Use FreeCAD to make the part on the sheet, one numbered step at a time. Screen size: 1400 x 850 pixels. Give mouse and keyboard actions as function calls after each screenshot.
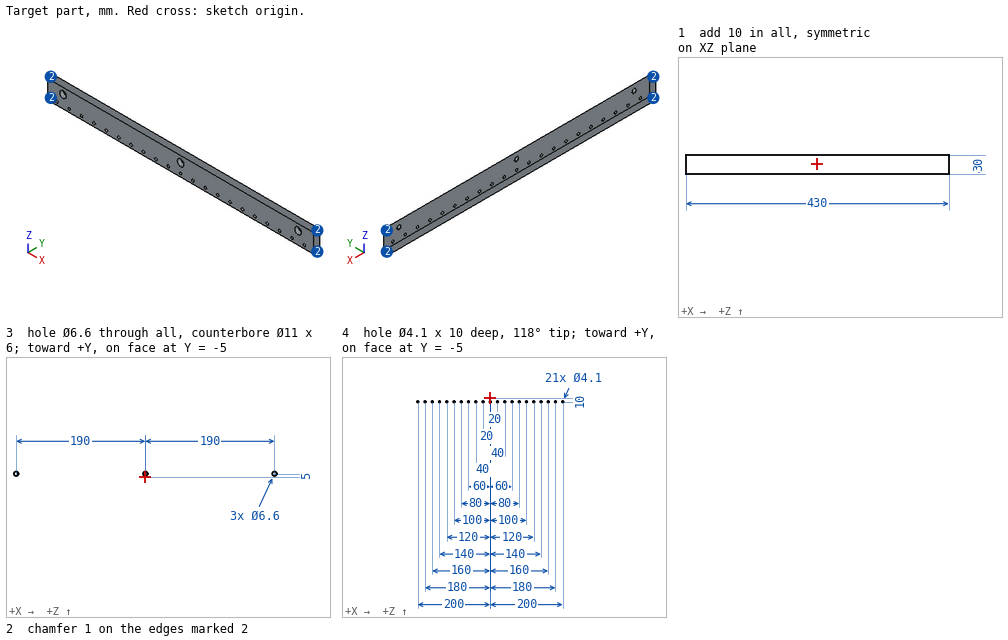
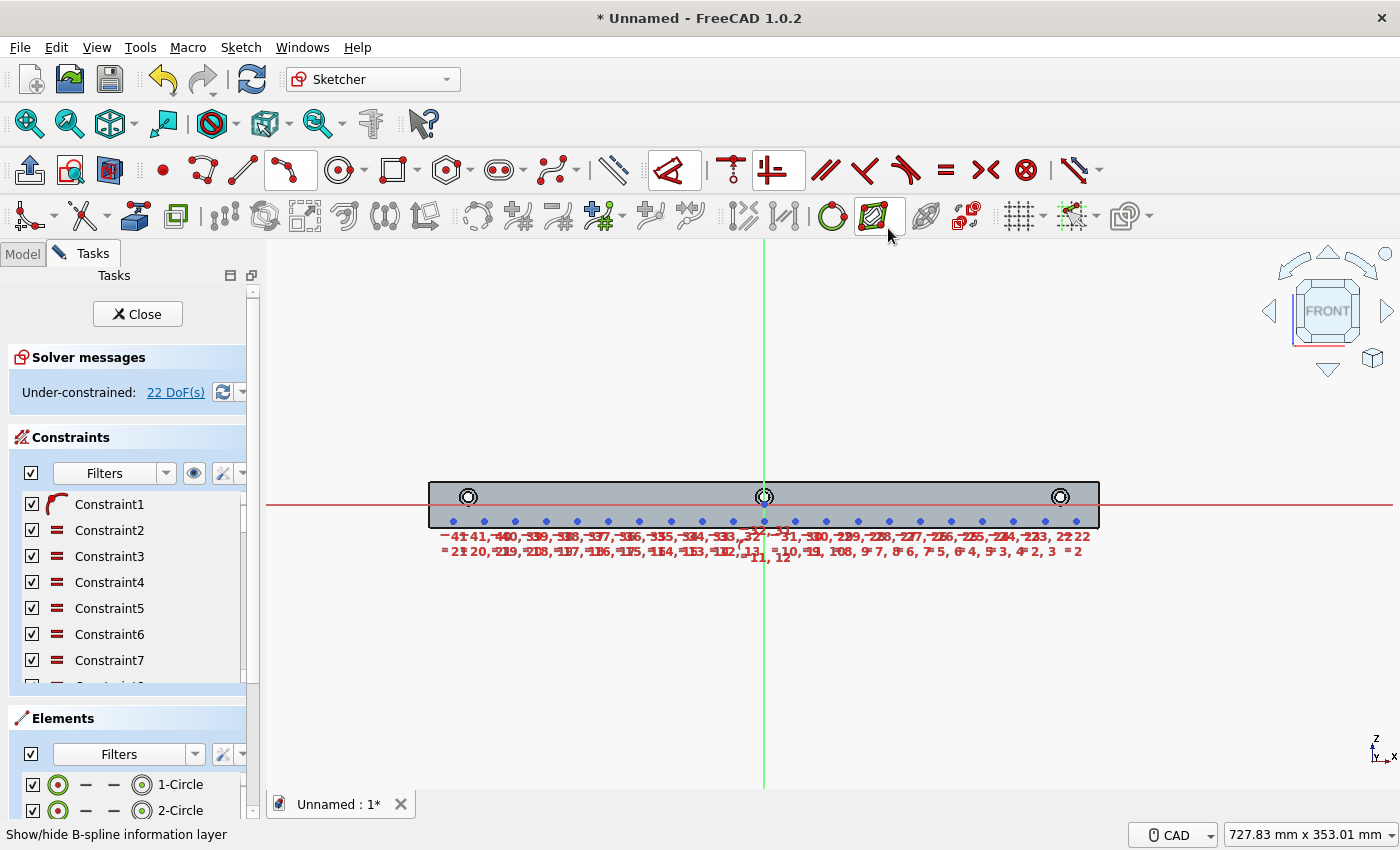
scroll(1074, 522, up, 10)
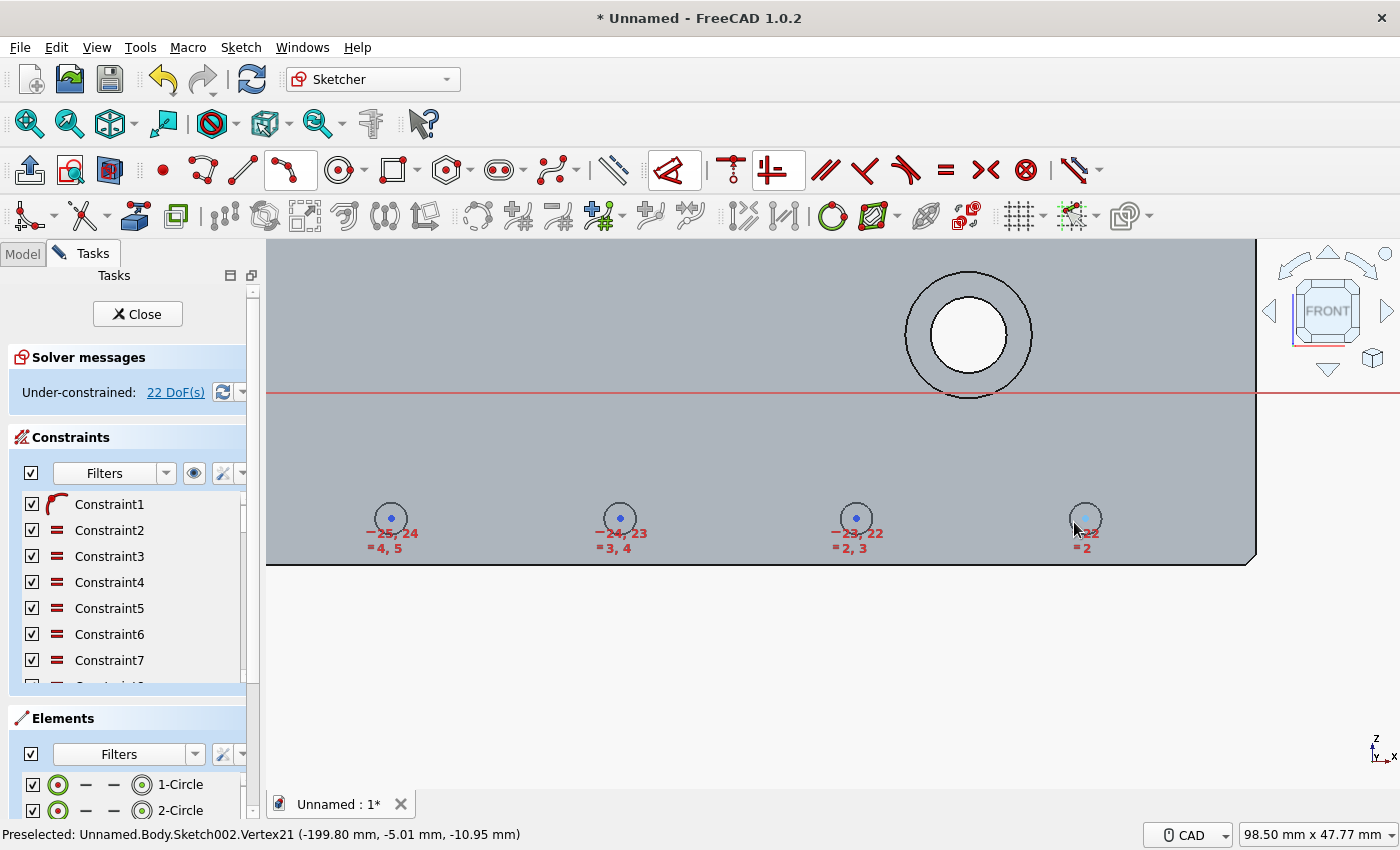
click(1070, 518)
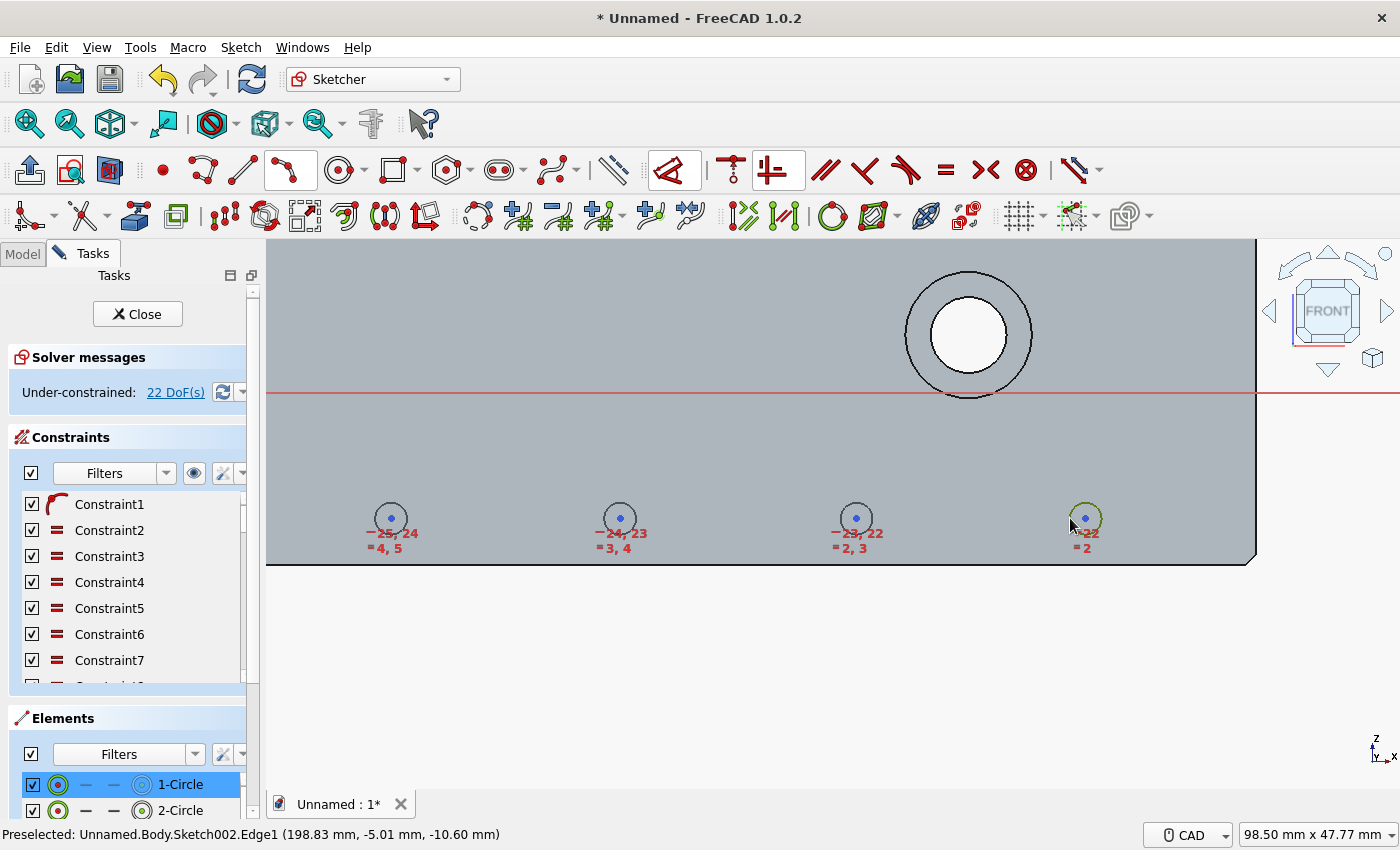
click(696, 170)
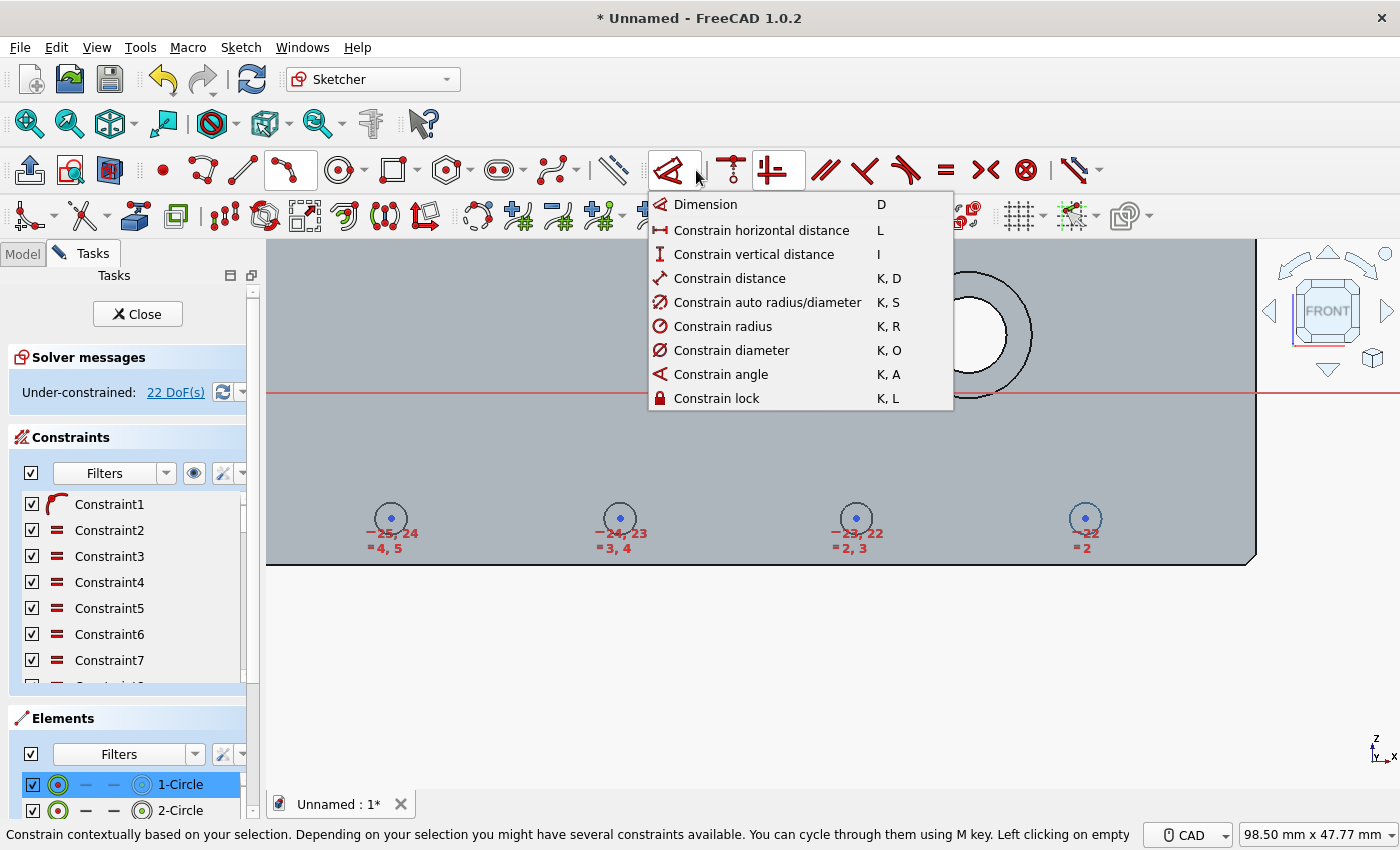
click(801, 350)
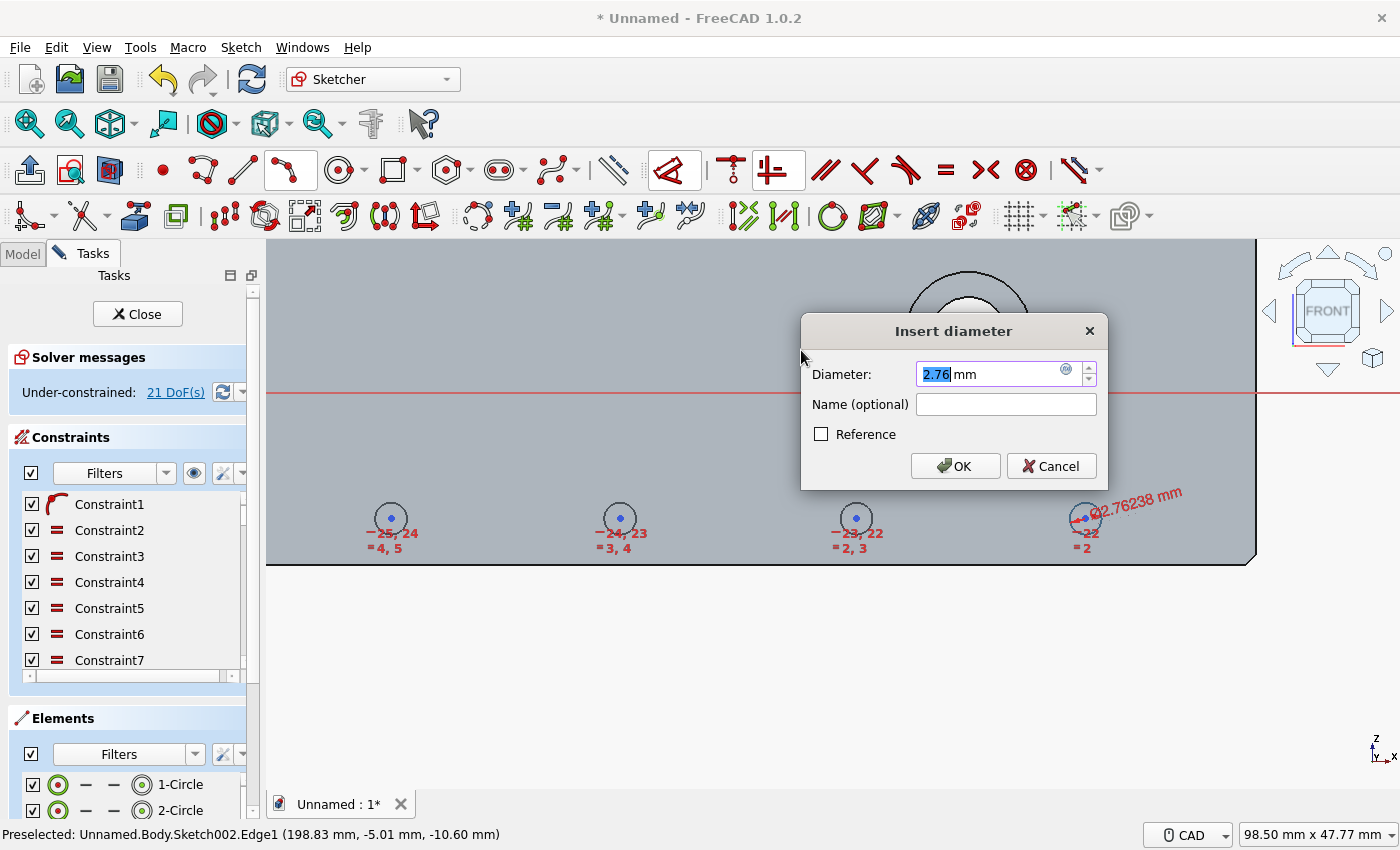
text(4.1)
key(Return)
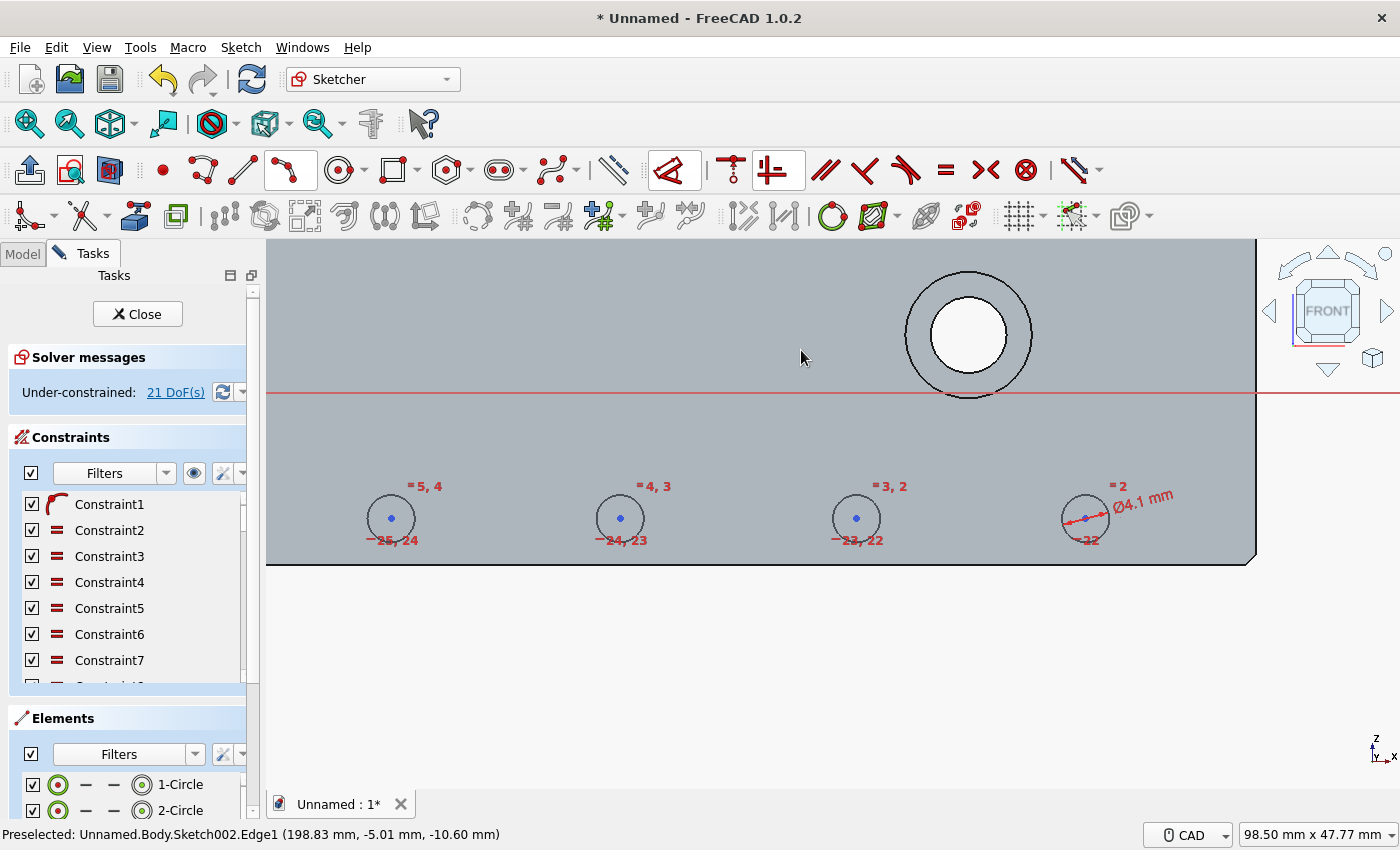
scroll(1075, 522, down, 10)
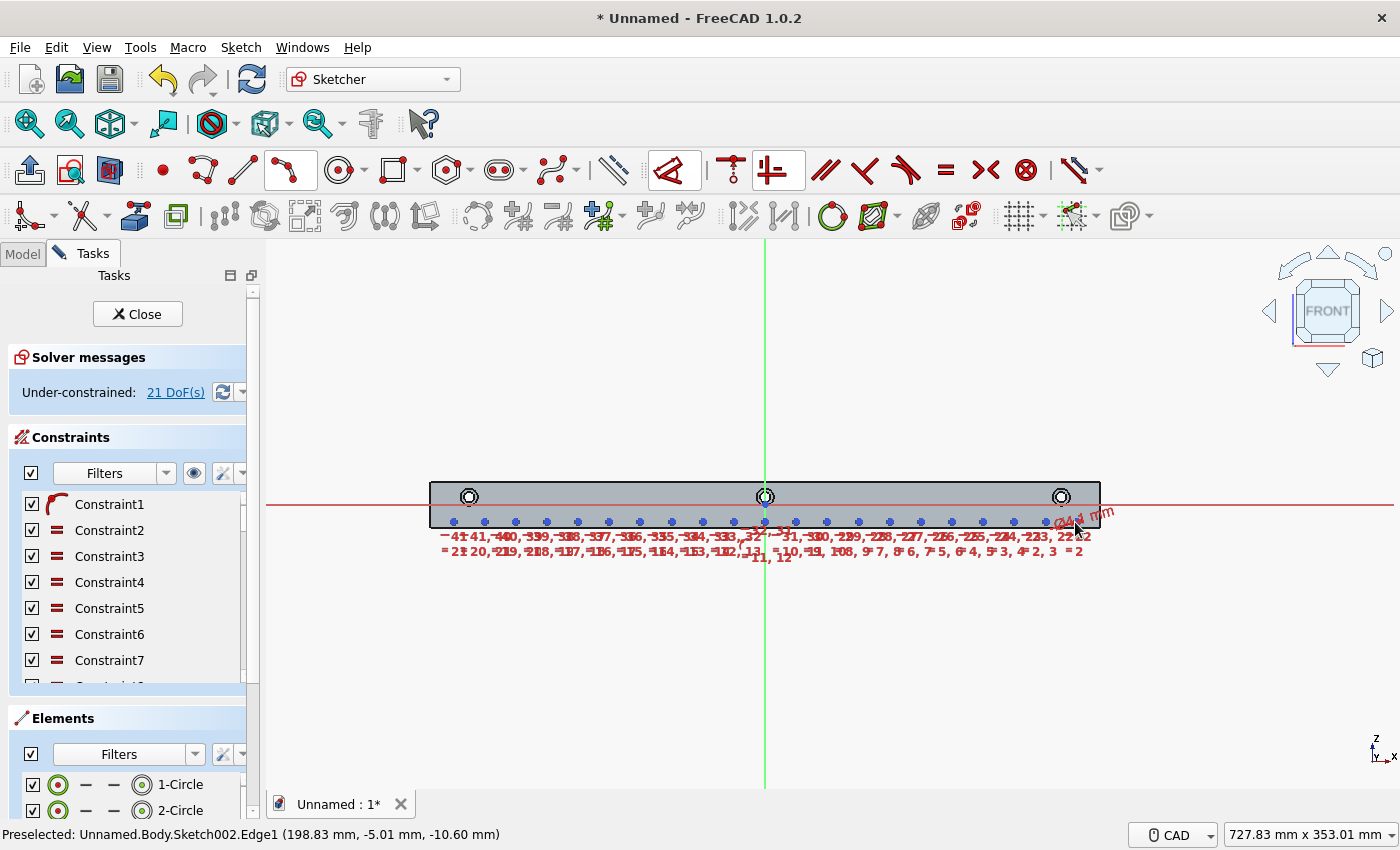
scroll(1077, 522, up, 5)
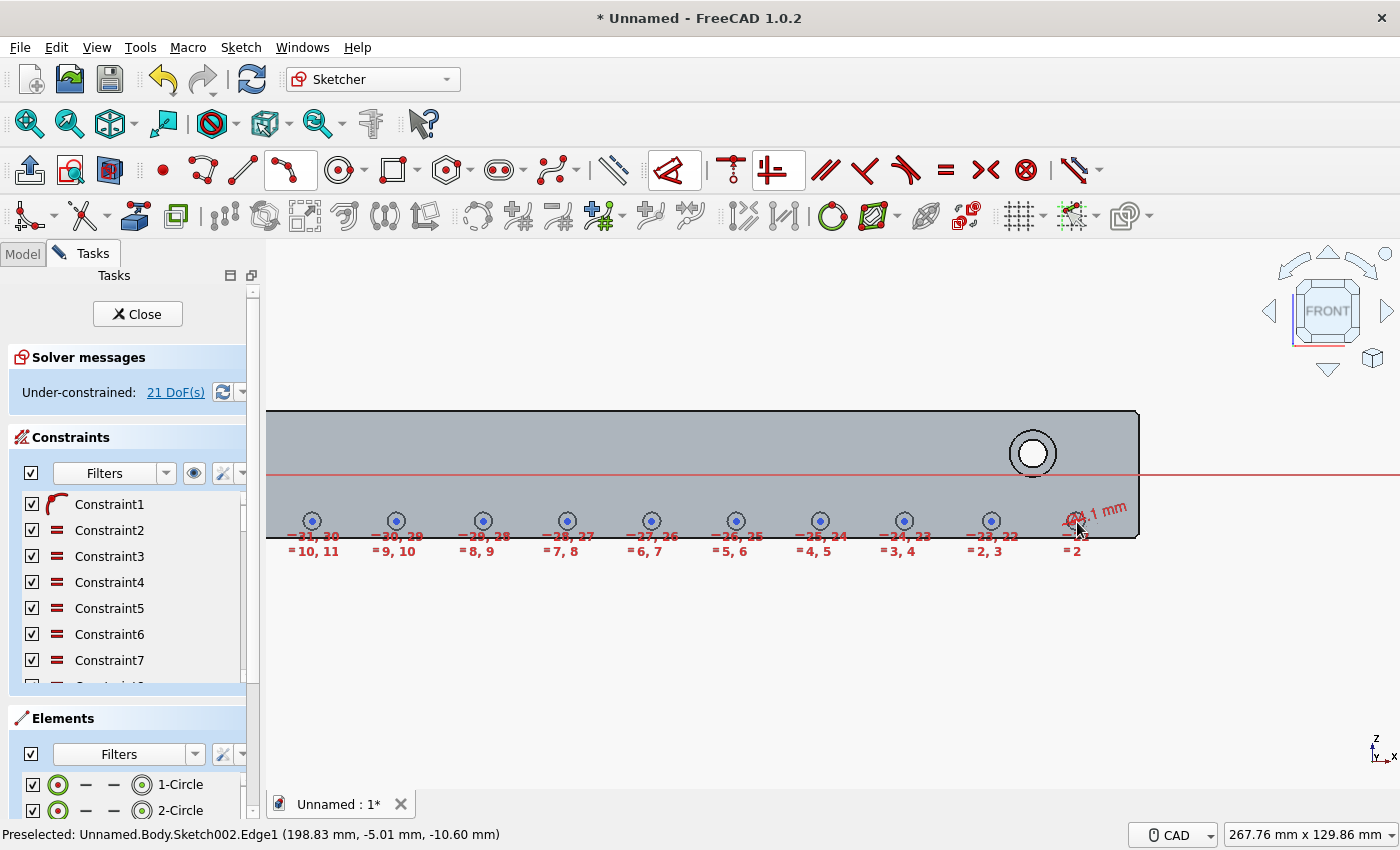
click(1076, 521)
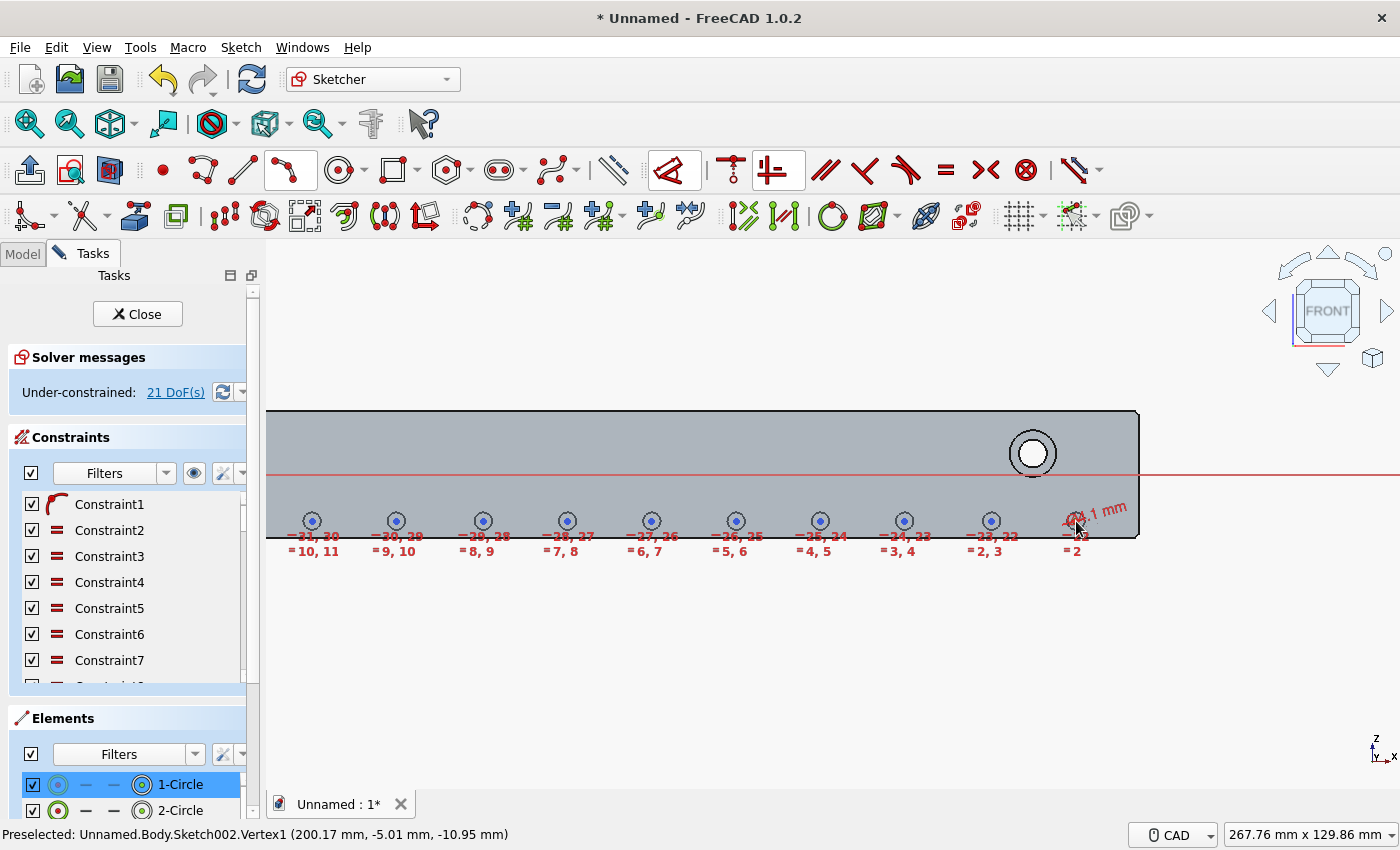
key(i)